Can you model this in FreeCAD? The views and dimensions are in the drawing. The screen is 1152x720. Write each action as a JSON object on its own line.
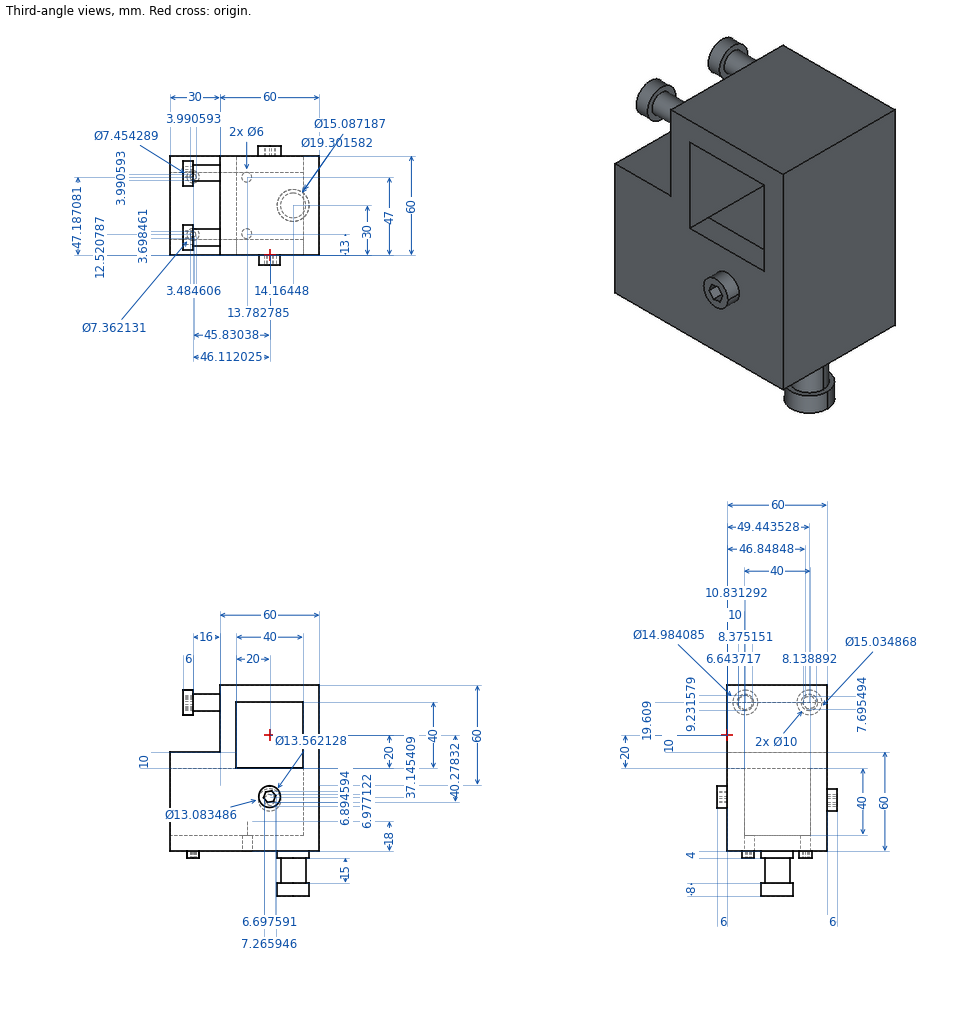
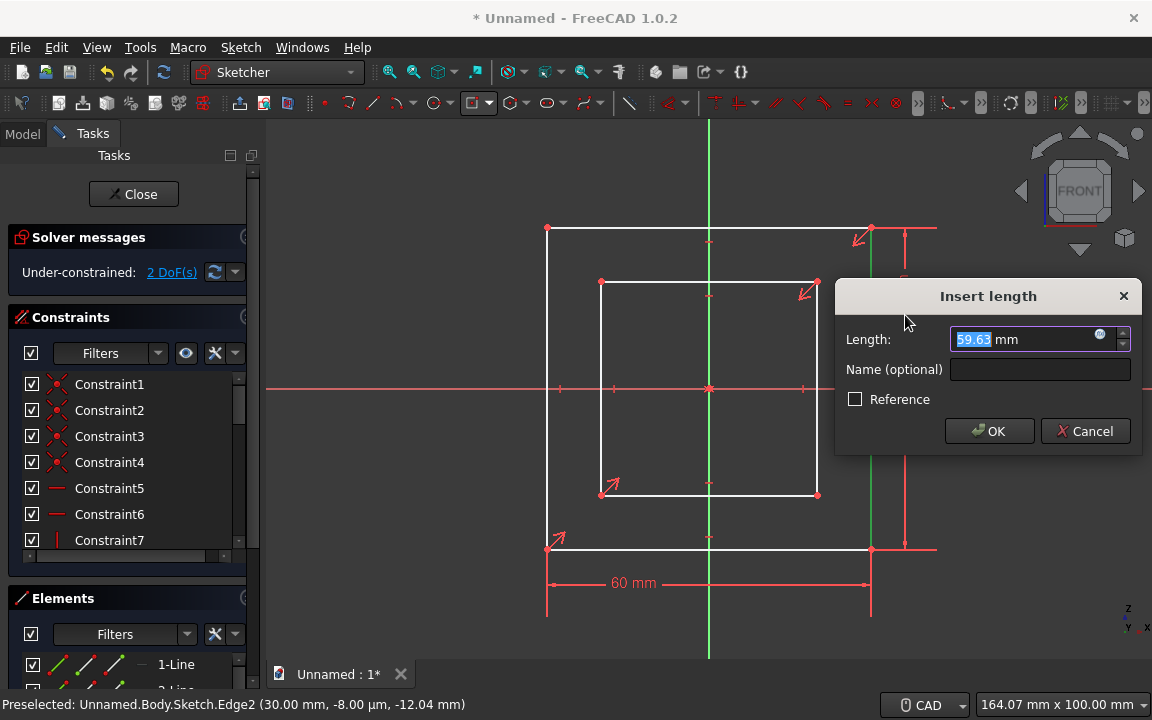
{"action": "type", "text": "60"}
{"action": "key", "text": "Return"}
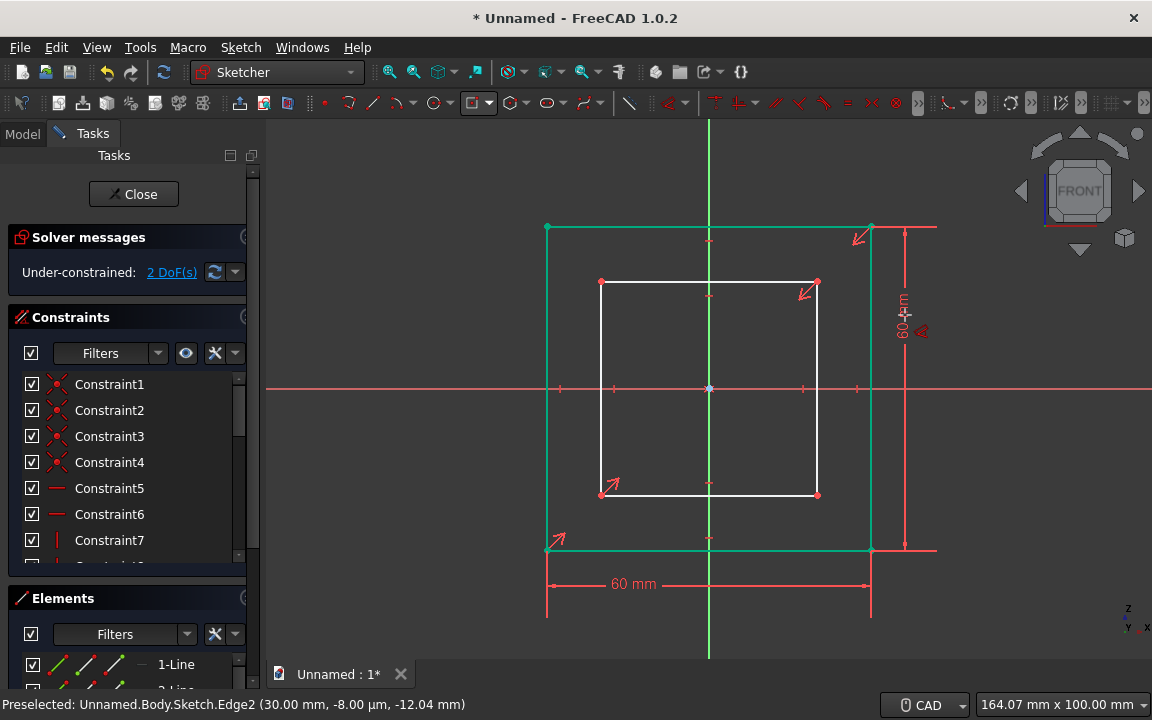
{"action": "left_click", "coordinate": [666, 496]}
{"action": "left_click", "coordinate": [659, 530]}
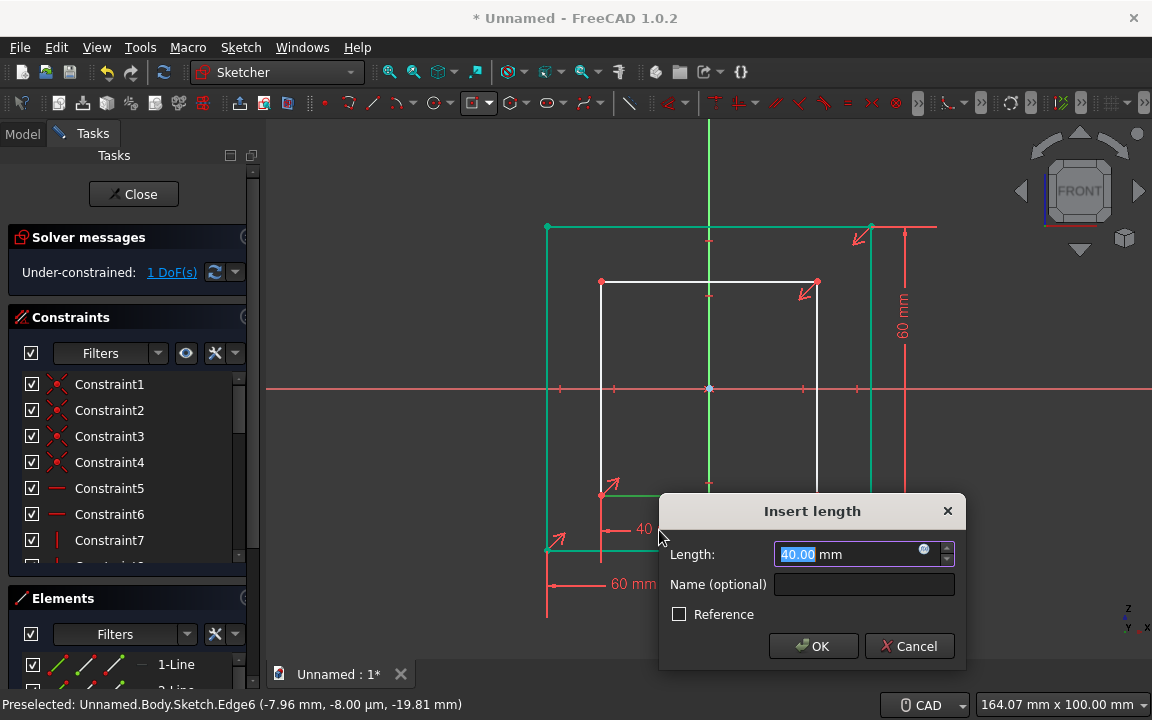
{"action": "type", "text": "40"}
{"action": "key", "text": "Return"}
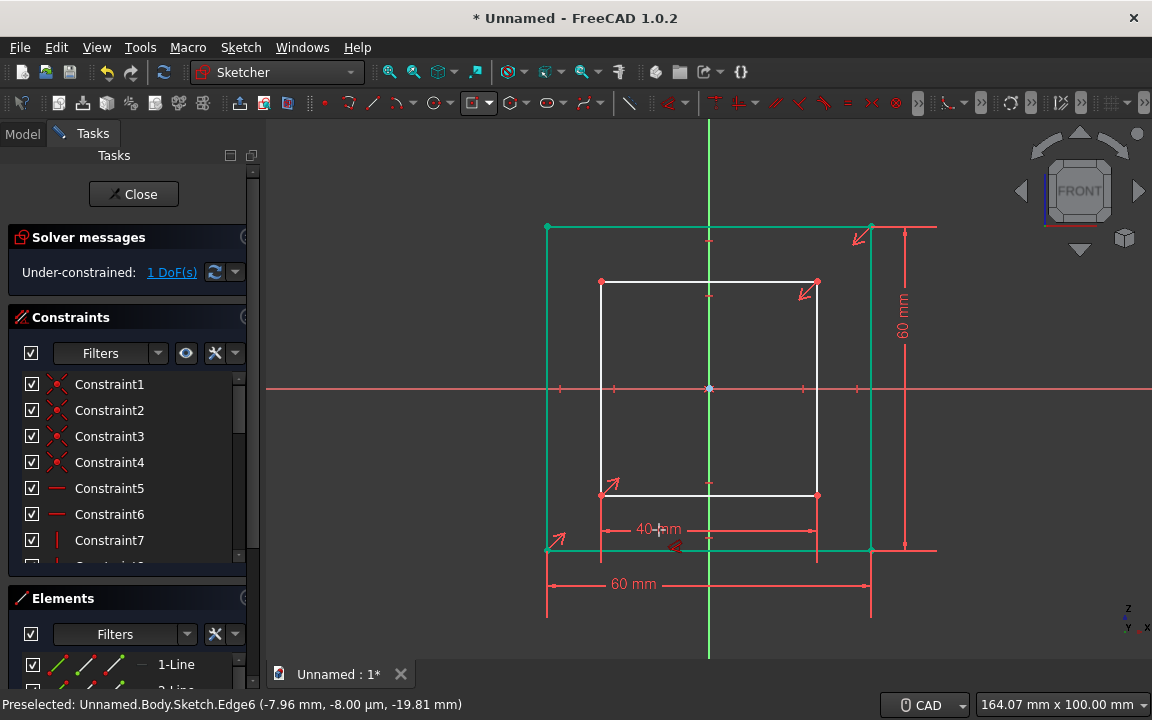
{"action": "left_click", "coordinate": [817, 432]}
{"action": "left_click", "coordinate": [851, 340]}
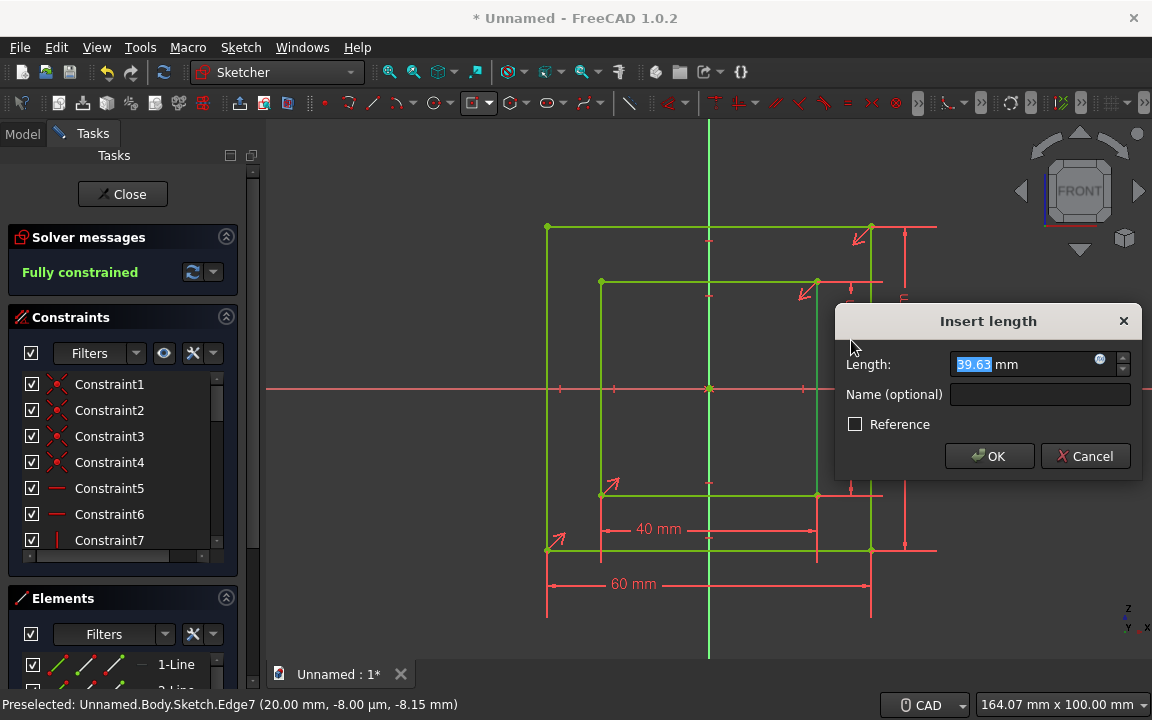
{"action": "type", "text": "40"}
{"action": "key", "text": "Return"}
{"action": "key", "text": "Escape"}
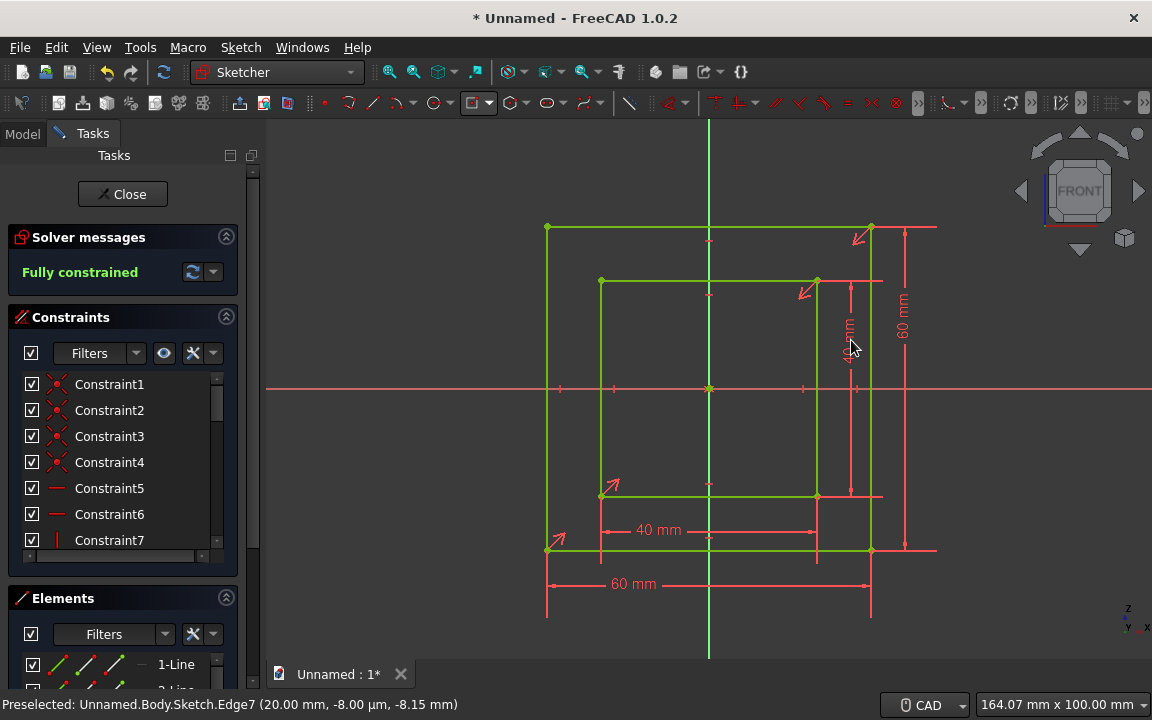
{"action": "left_click", "coordinate": [123, 194]}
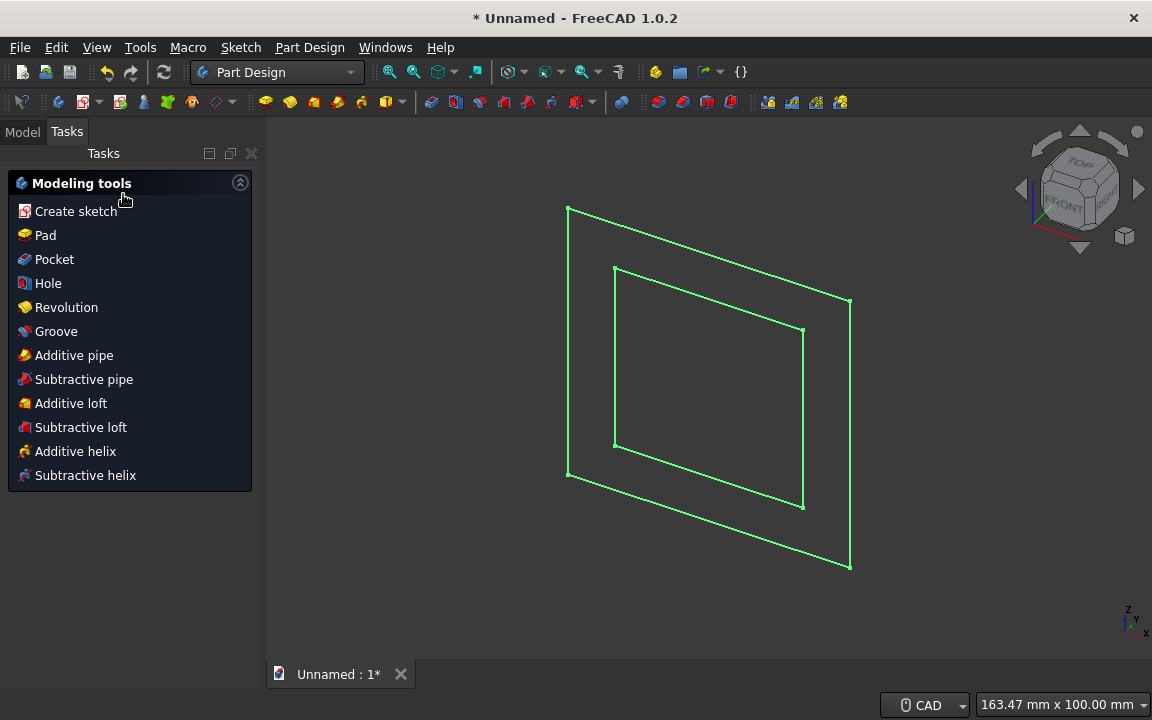
{"action": "left_click", "coordinate": [266, 102]}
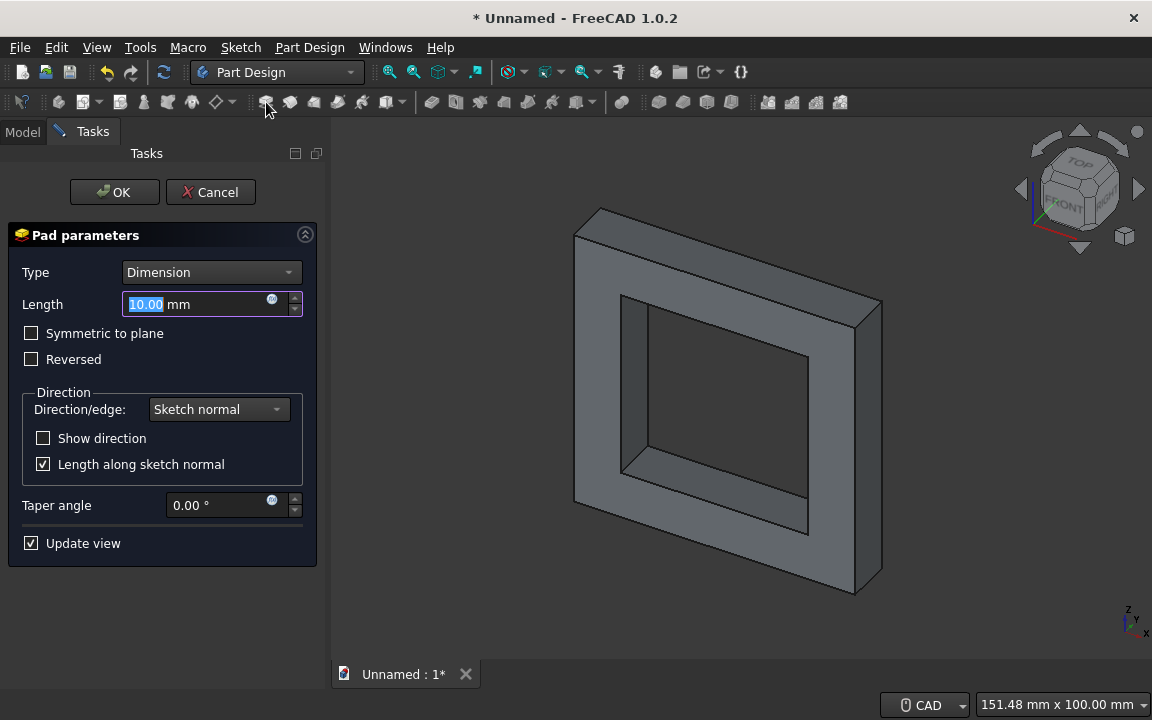
{"action": "type", "text": "60"}
{"action": "key", "text": "Tab"}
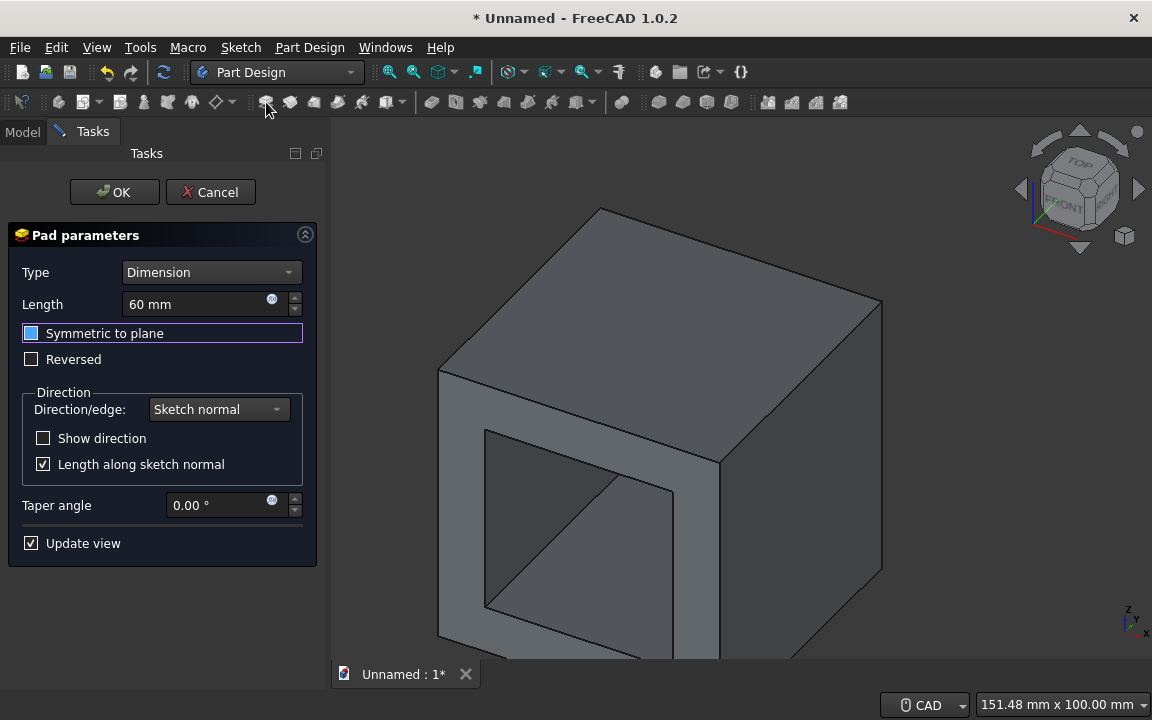
{"action": "left_click", "coordinate": [30, 359]}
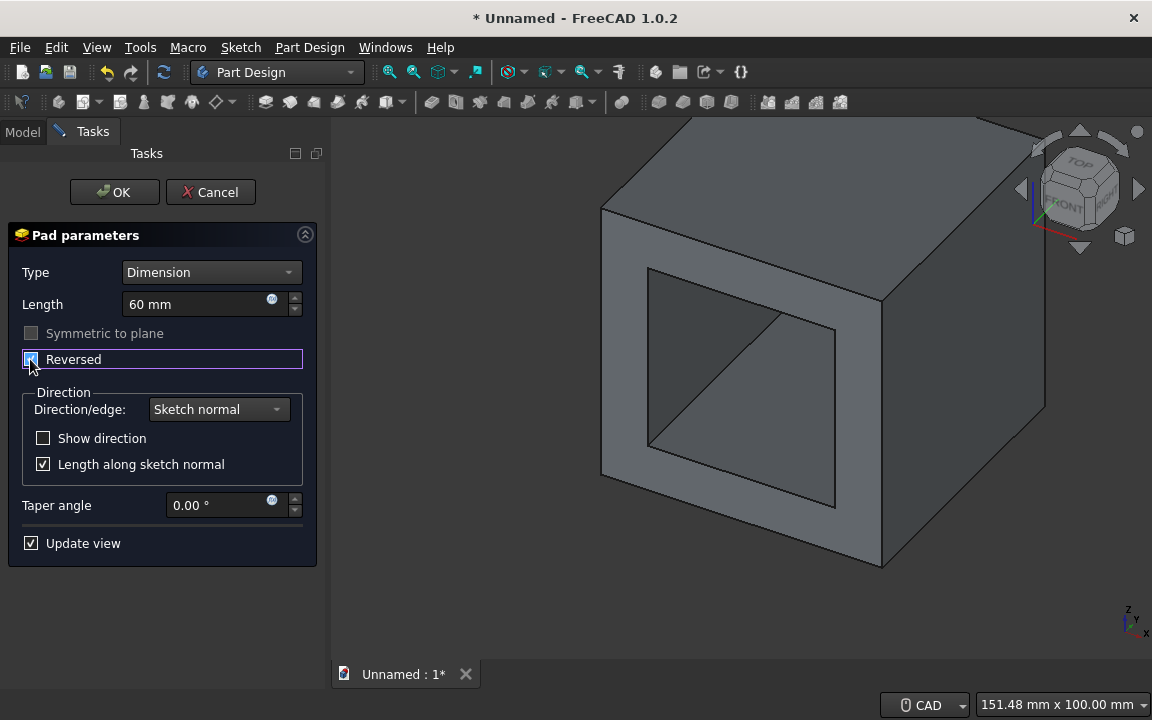
{"action": "left_click", "coordinate": [115, 192]}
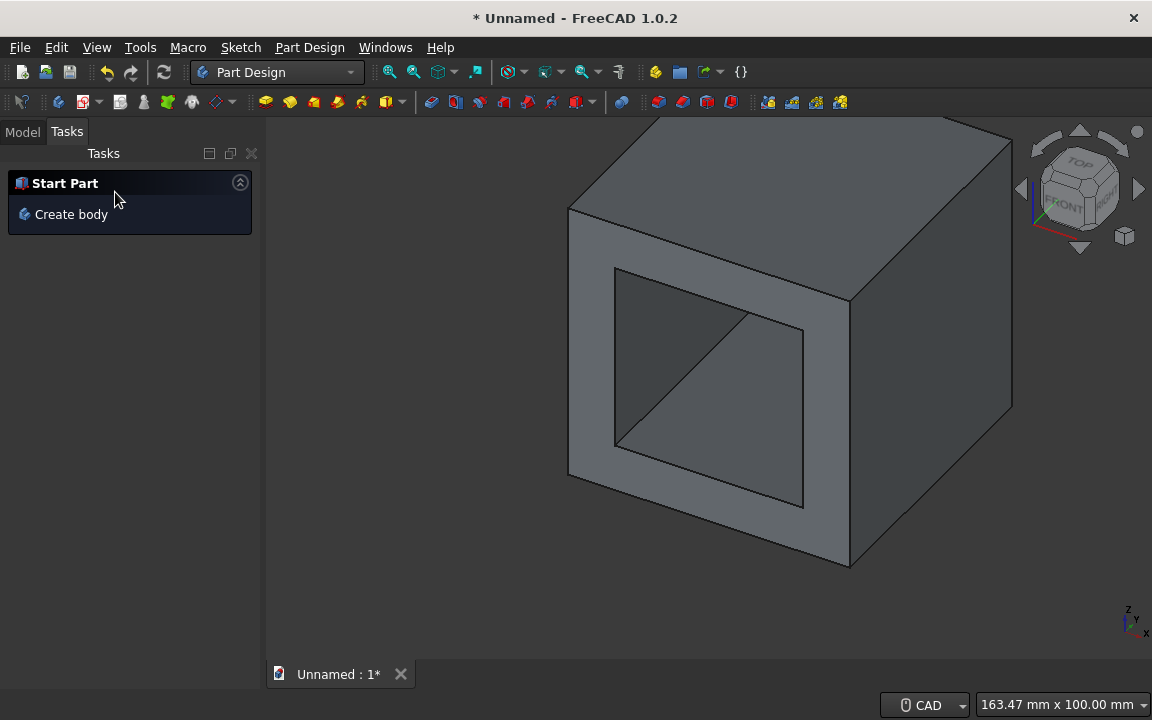
{"action": "left_click", "coordinate": [390, 72]}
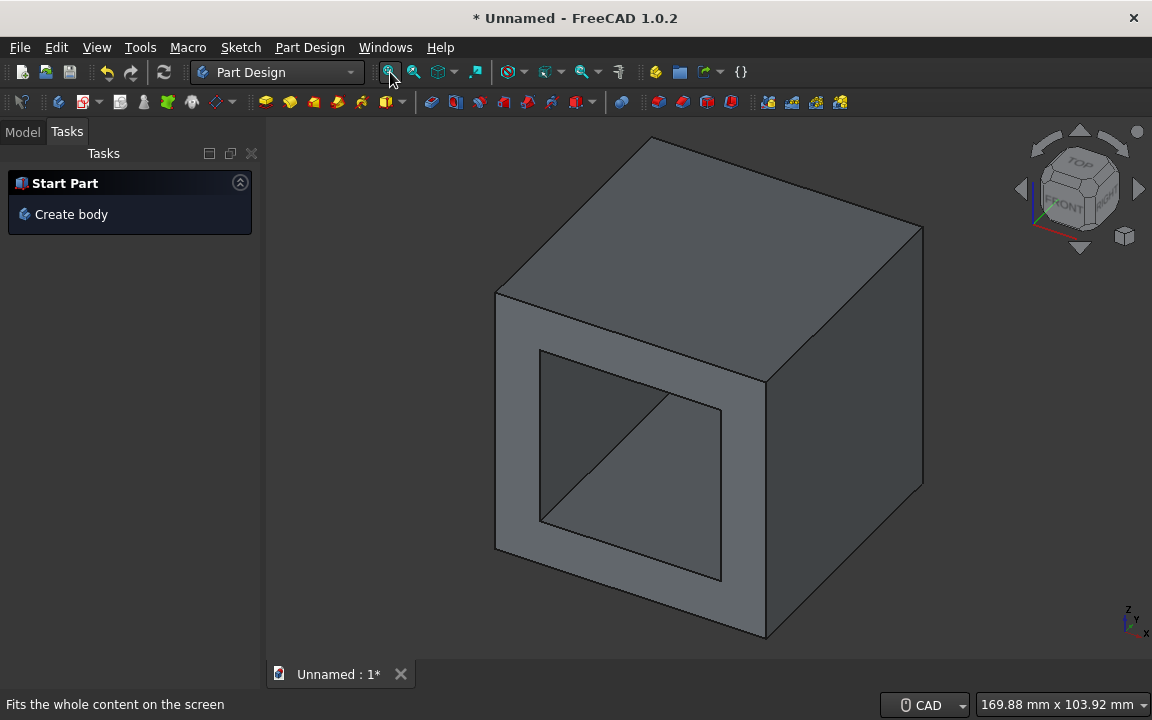
{"action": "key", "text": "6"}